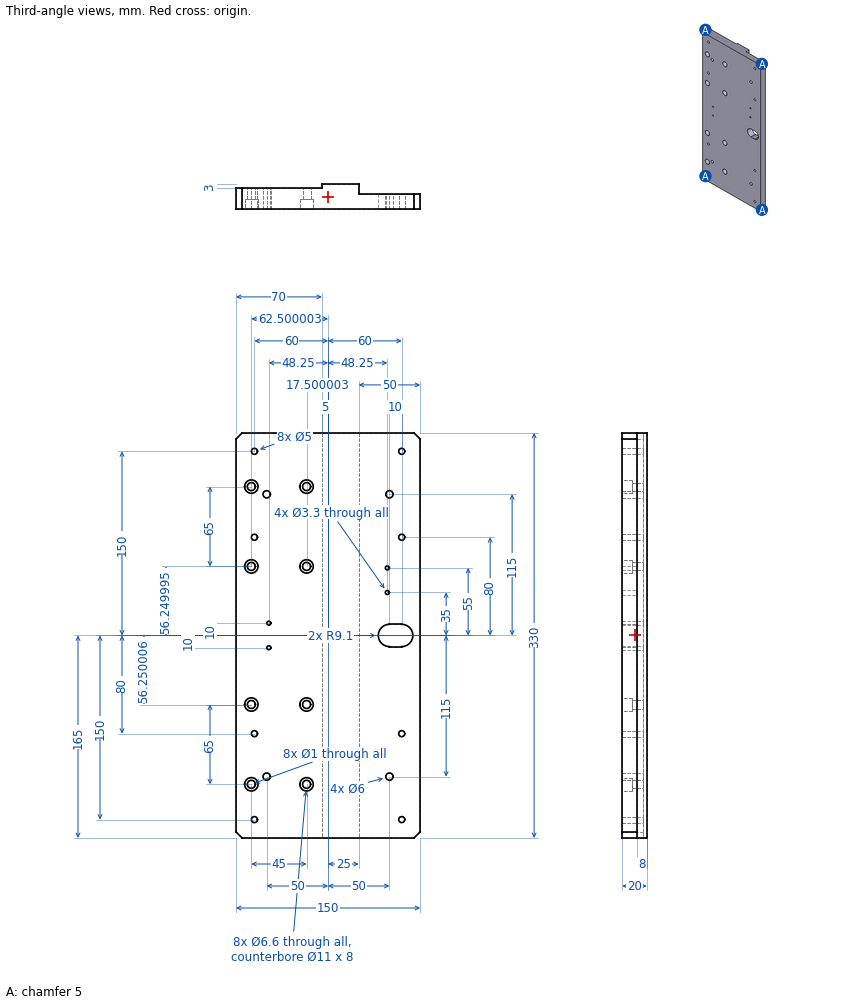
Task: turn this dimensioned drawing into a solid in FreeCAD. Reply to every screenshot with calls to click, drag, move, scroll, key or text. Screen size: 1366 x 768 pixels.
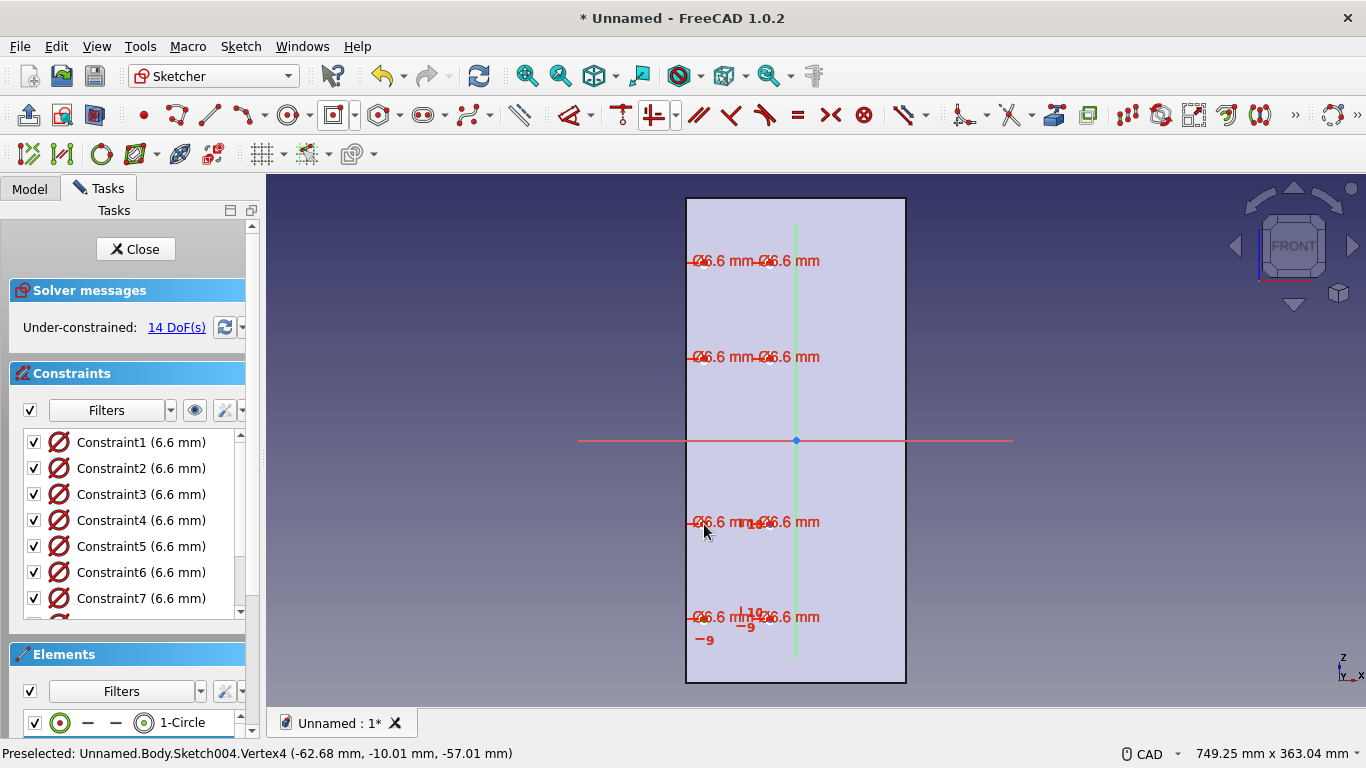
key(v)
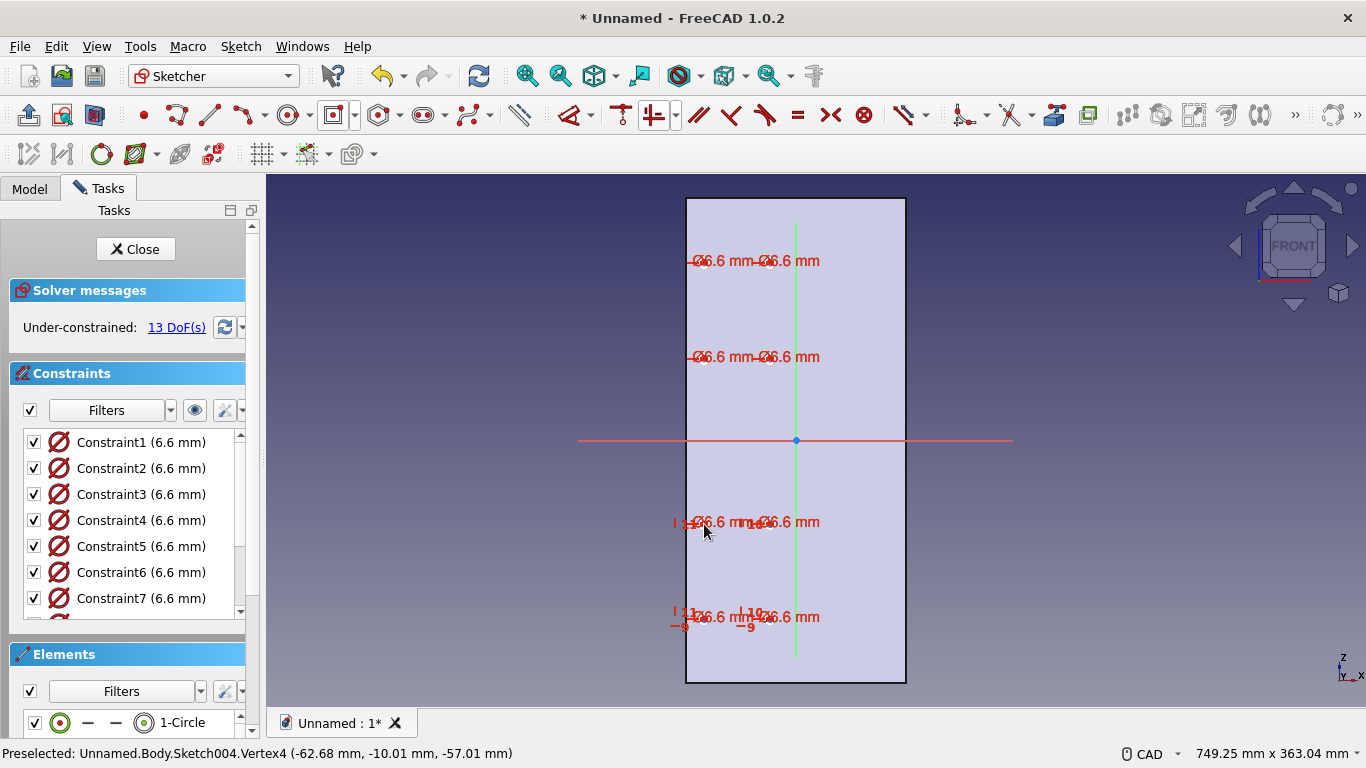
click(770, 524)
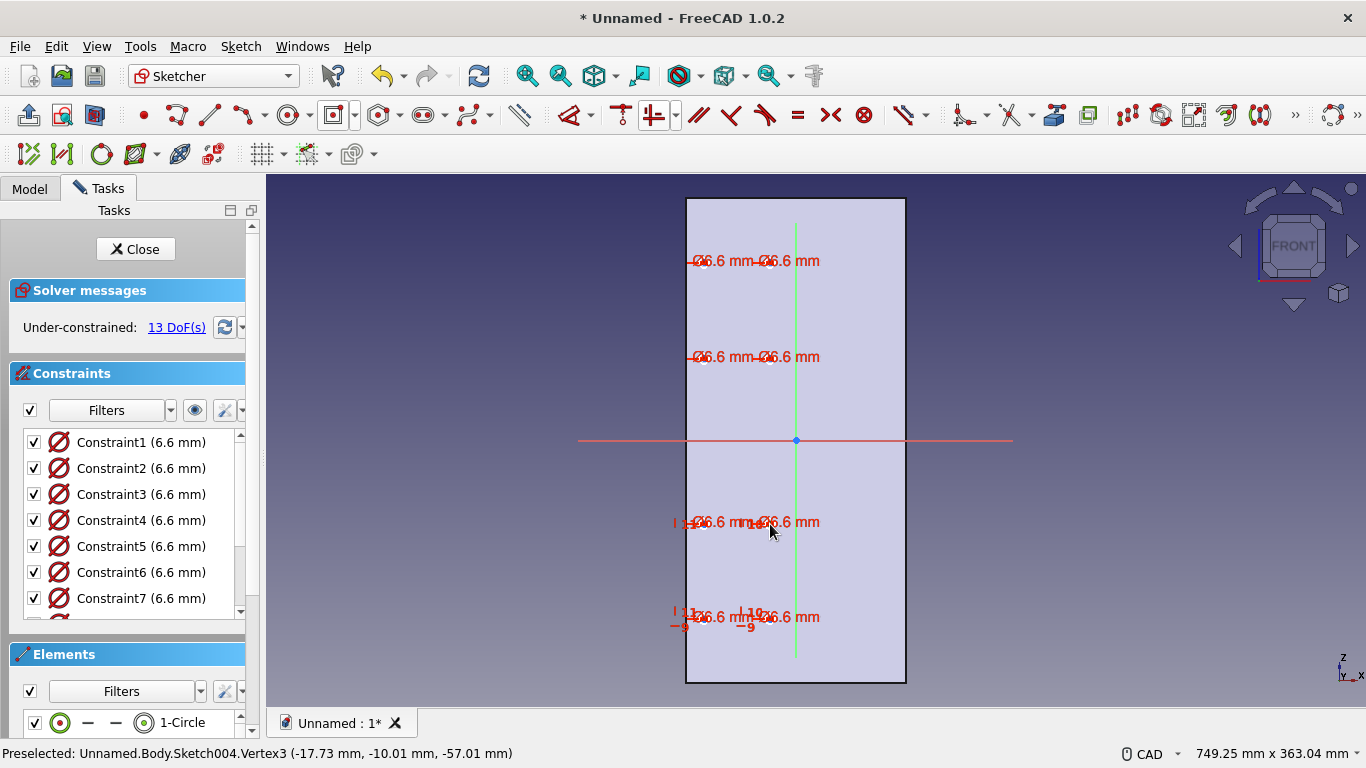
click(704, 524)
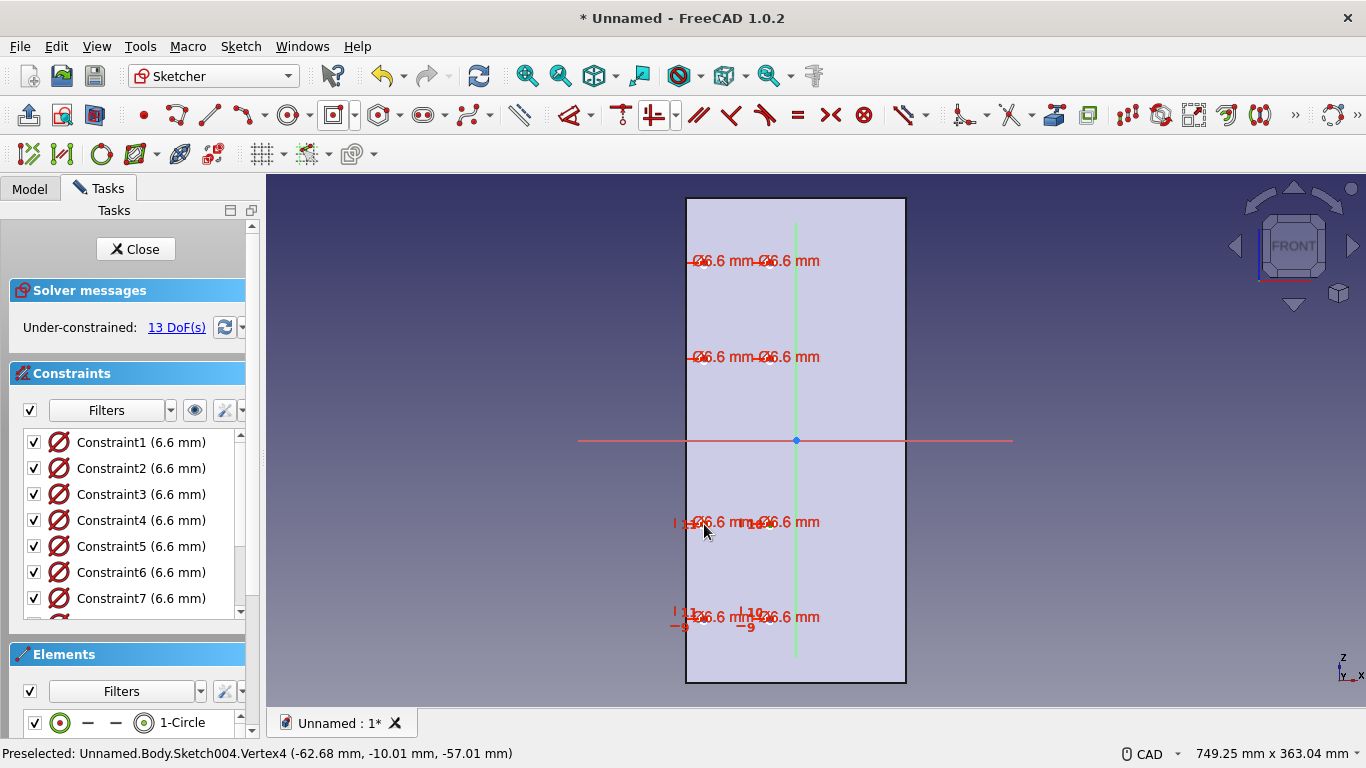
key(h)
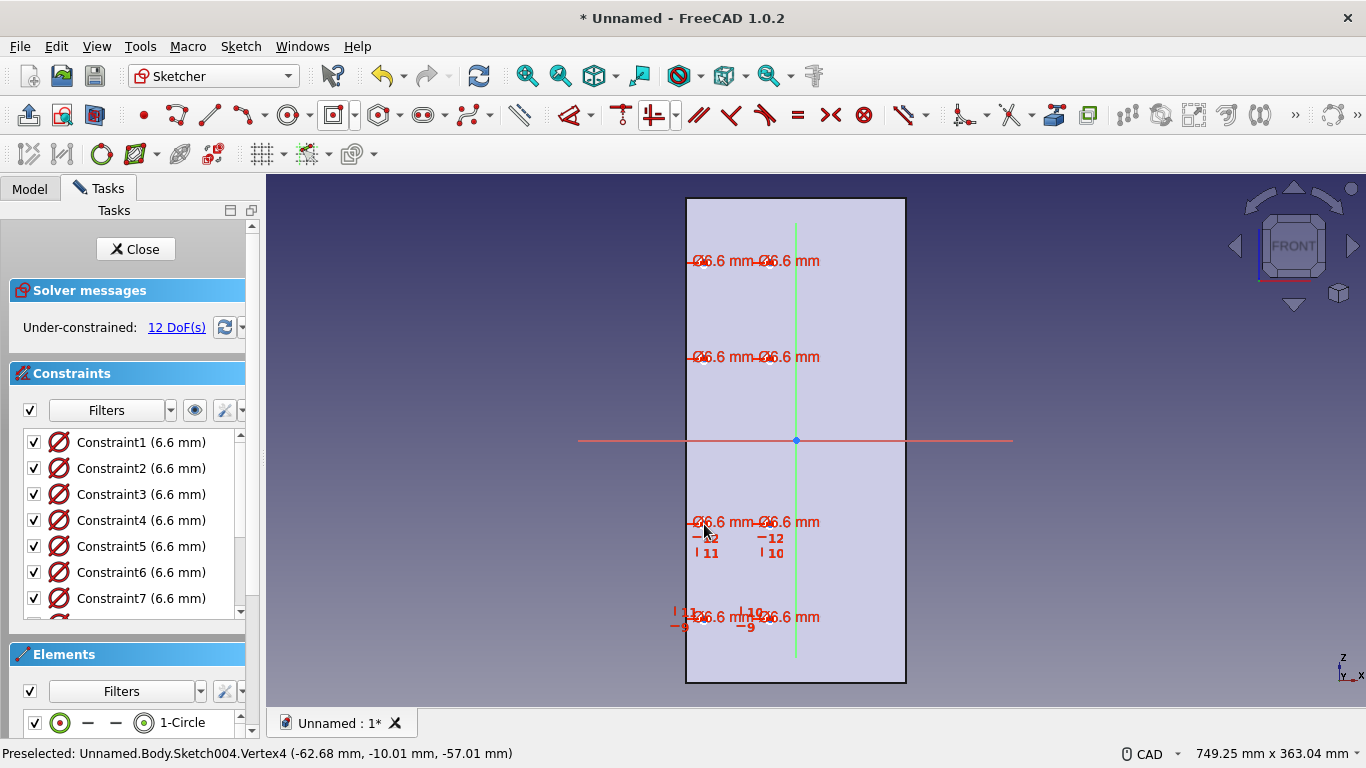
click(770, 359)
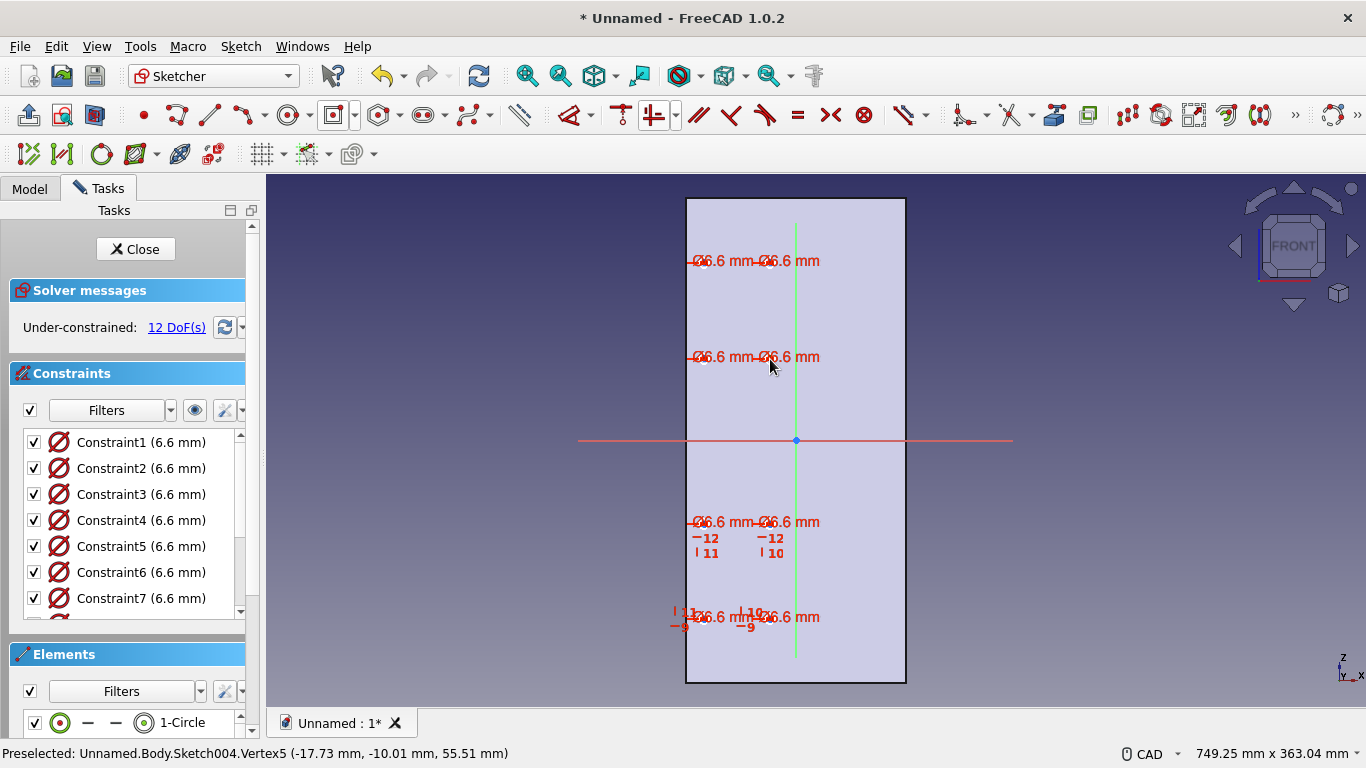
click(704, 359)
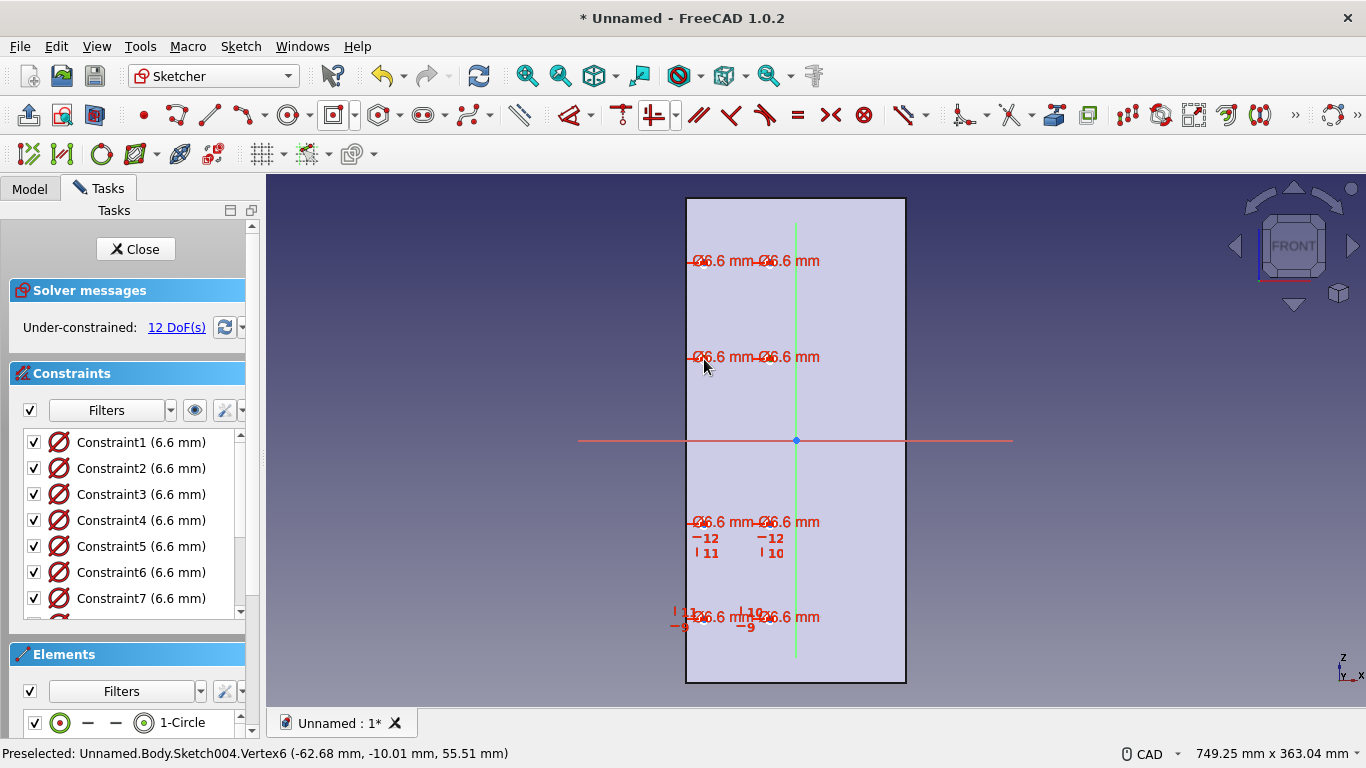
click(676, 116)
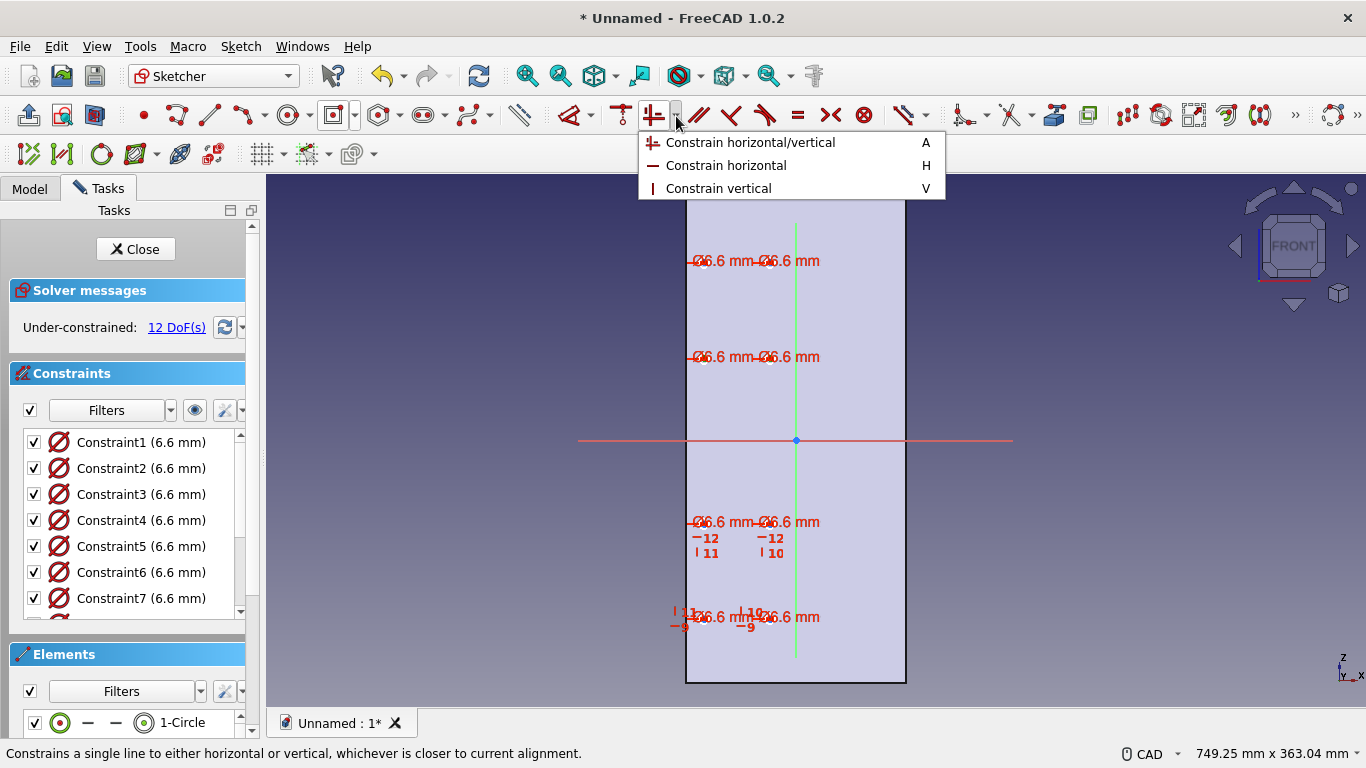
click(792, 166)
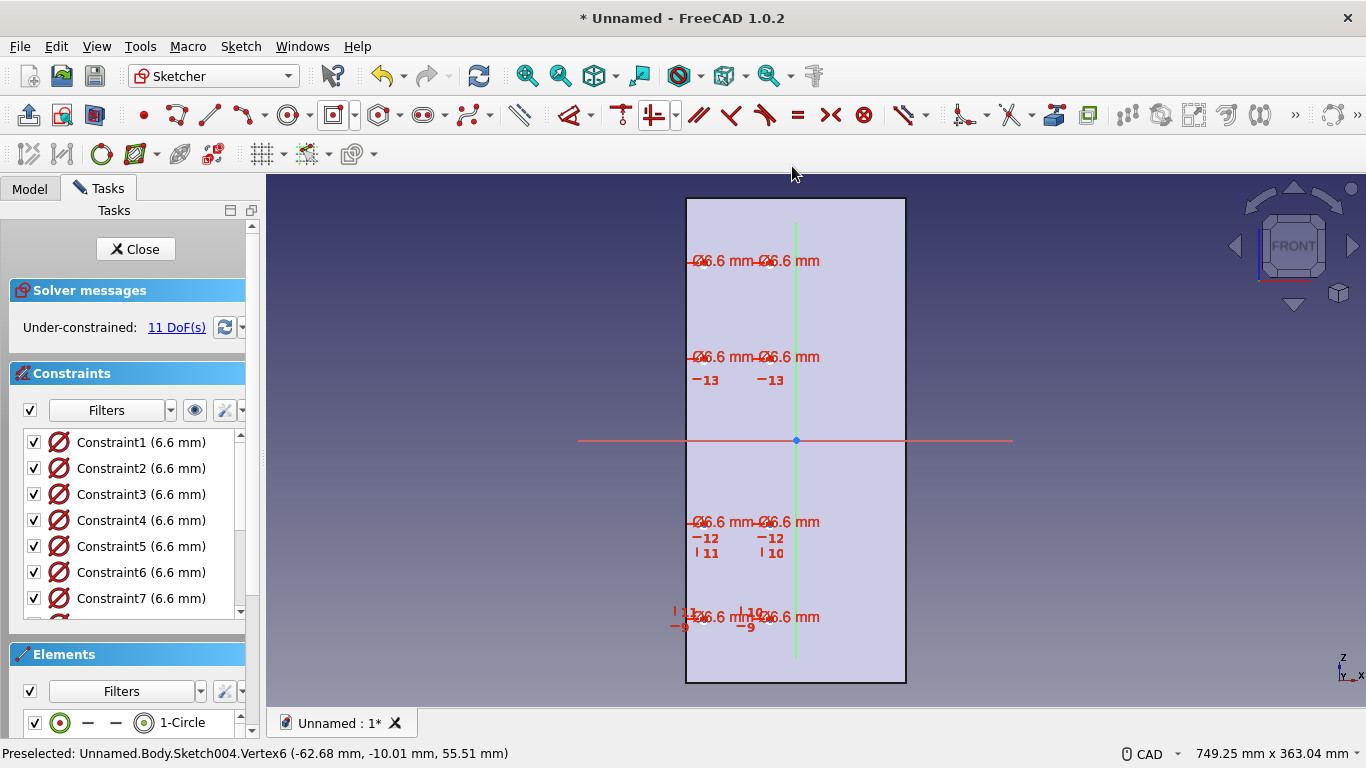
click(770, 359)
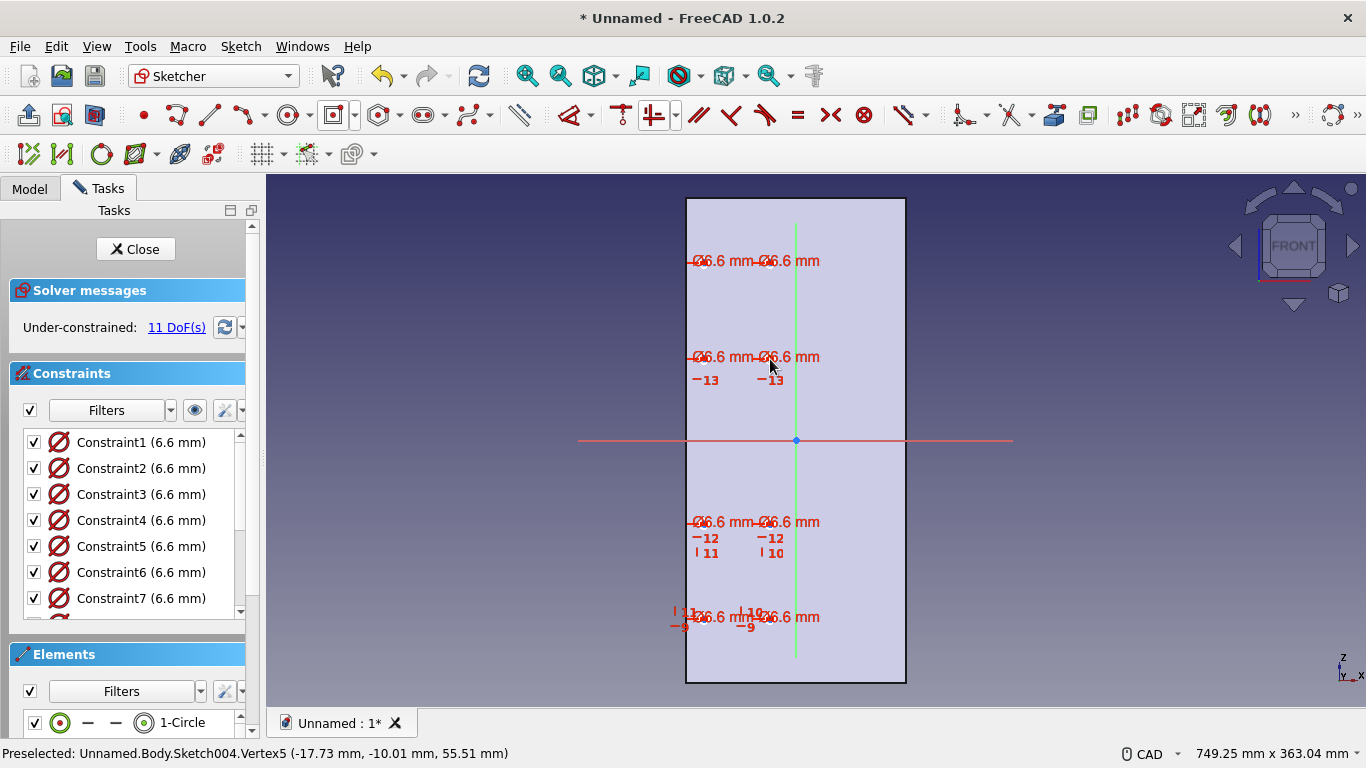
click(770, 263)